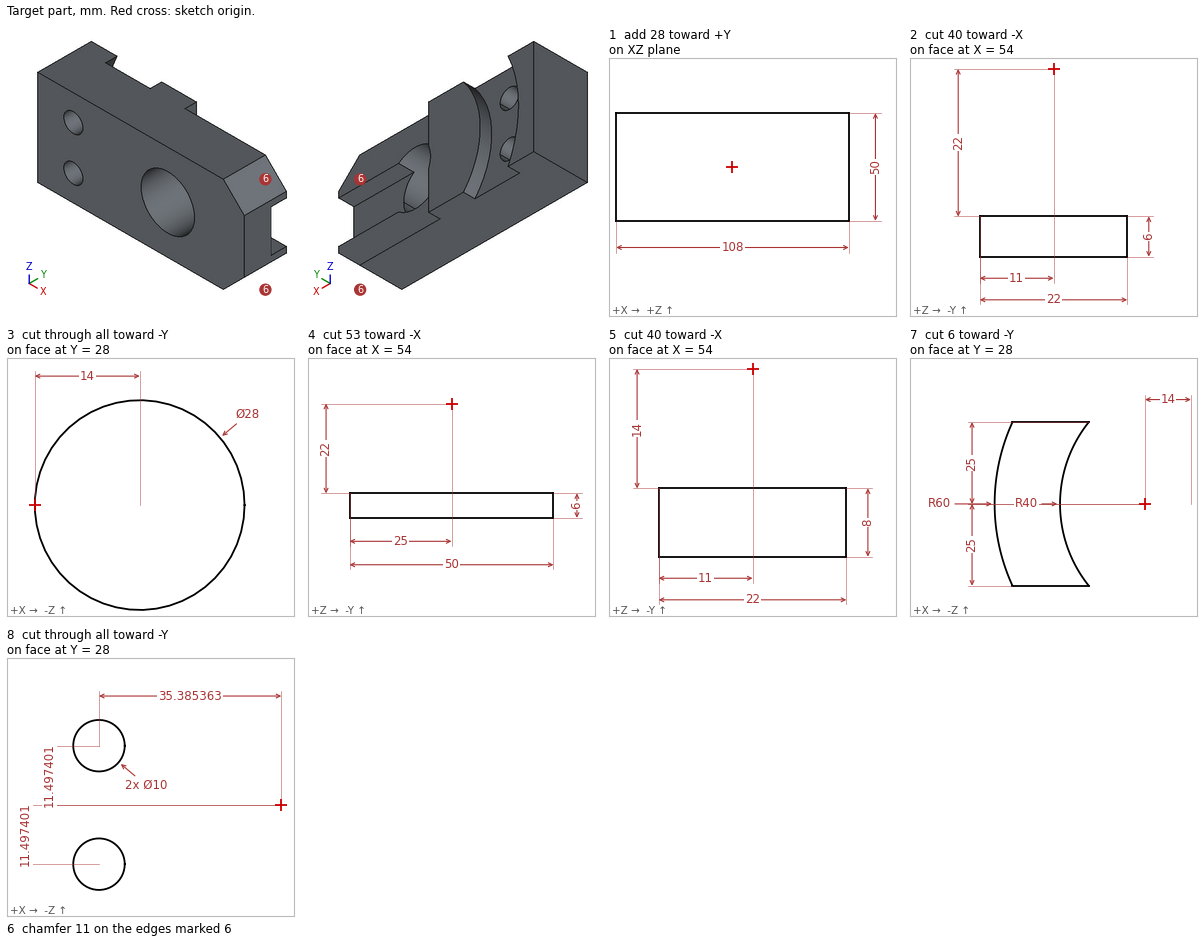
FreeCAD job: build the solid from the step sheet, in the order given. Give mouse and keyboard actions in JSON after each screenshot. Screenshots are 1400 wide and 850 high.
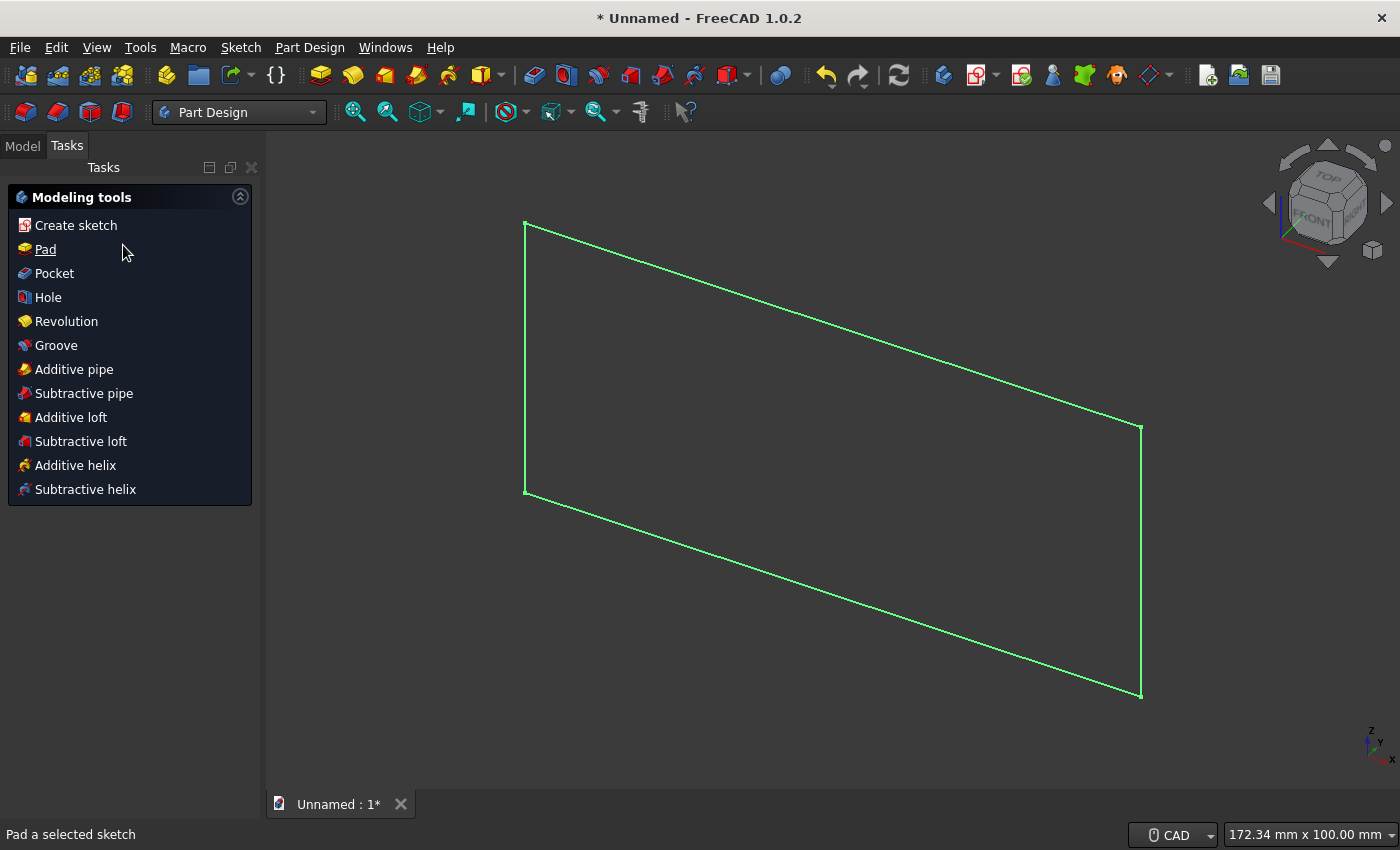
{"action": "left_click", "coordinate": [322, 76]}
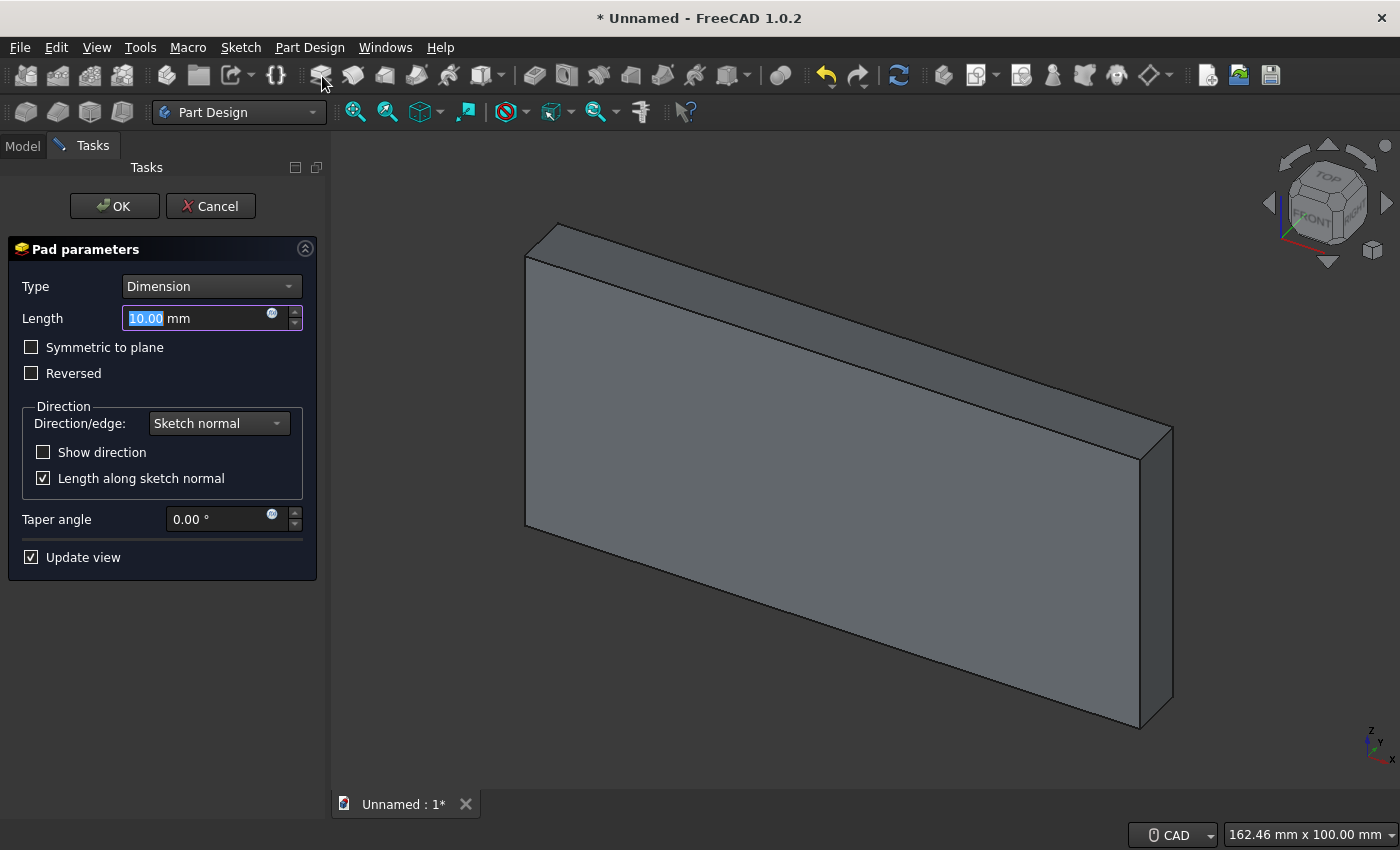
{"action": "type", "text": "28"}
{"action": "key", "text": "Tab"}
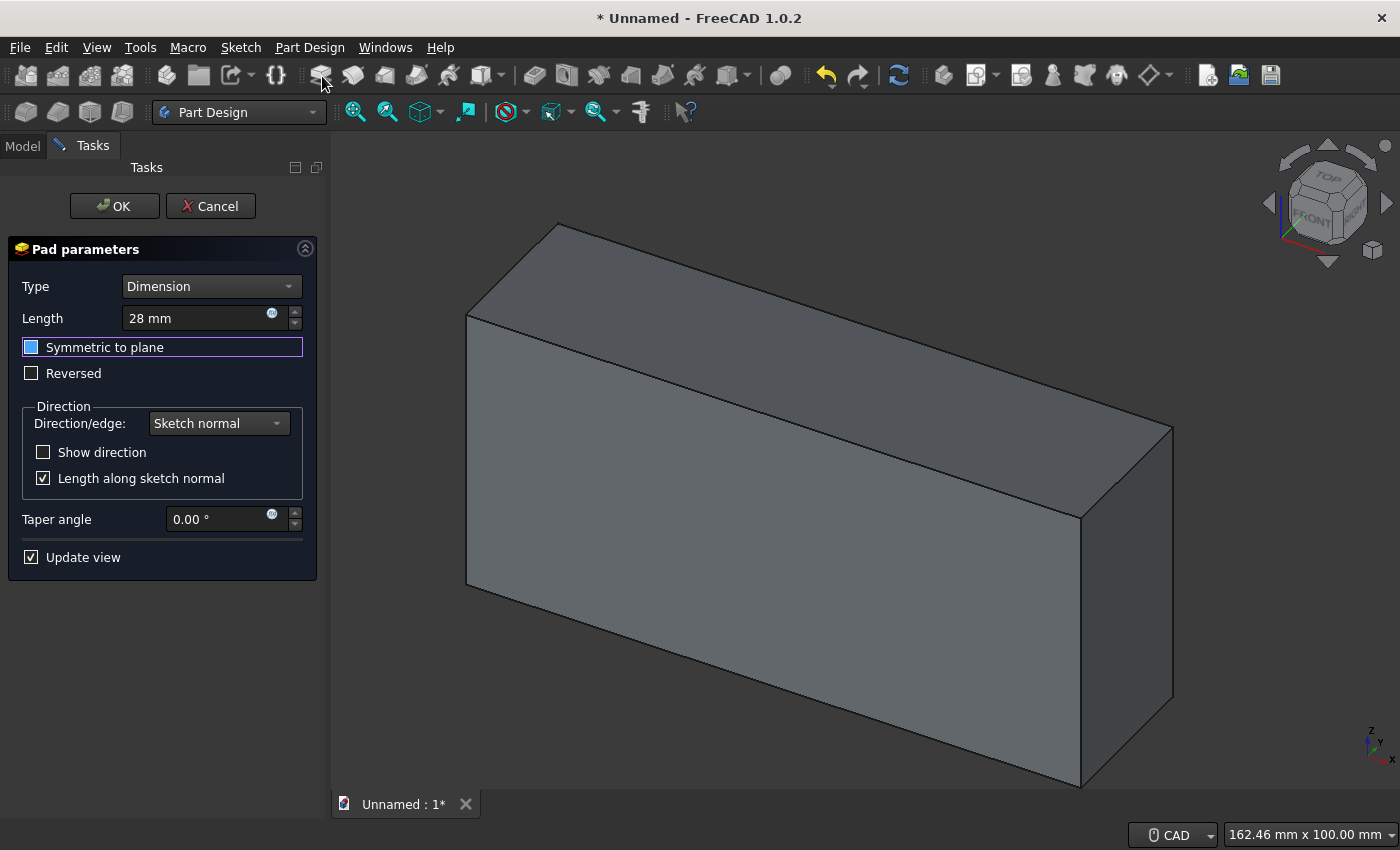
{"action": "left_click", "coordinate": [30, 373]}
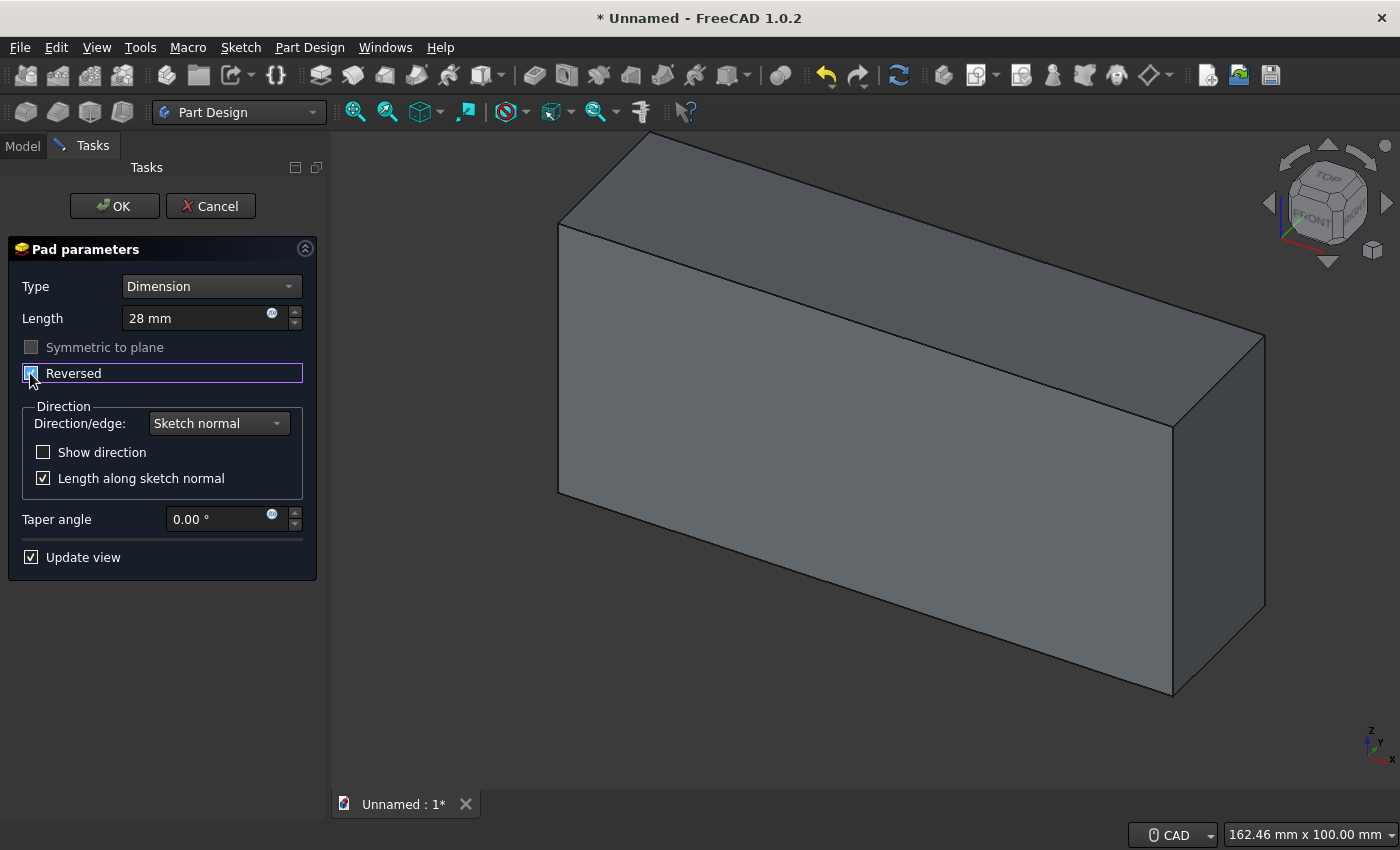
{"action": "left_click", "coordinate": [115, 206]}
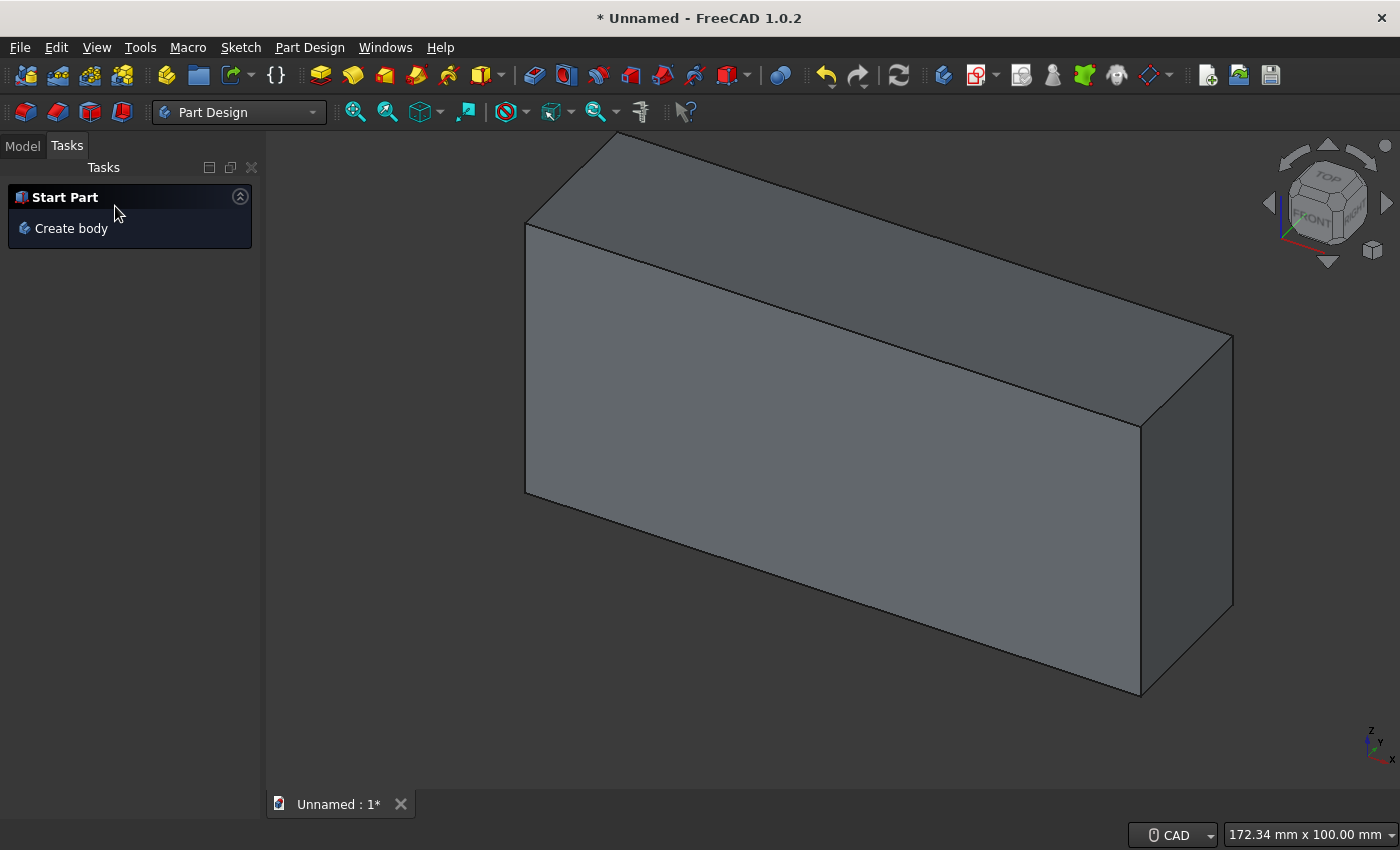
{"action": "left_click", "coordinate": [1187, 515]}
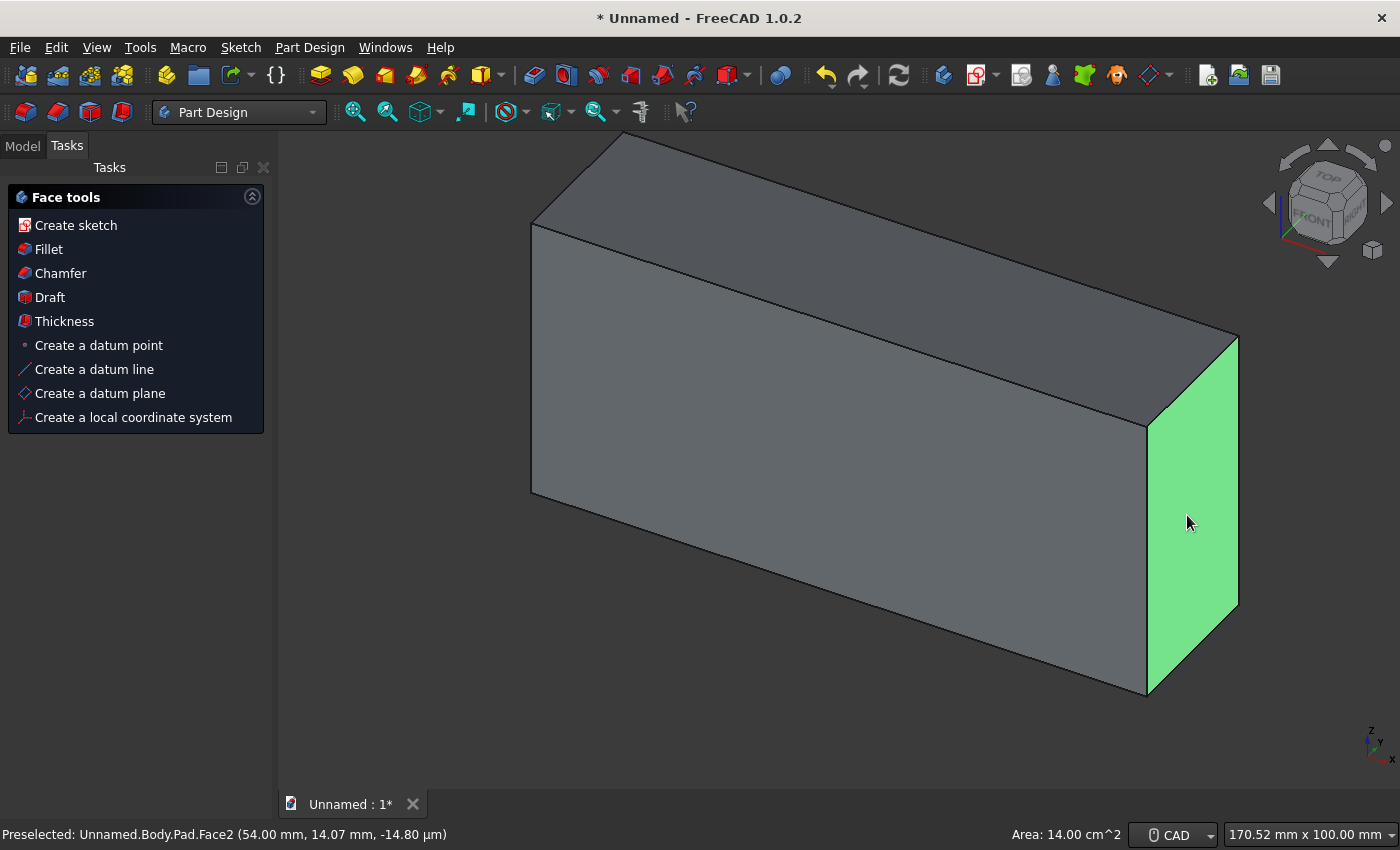
{"action": "left_click", "coordinate": [976, 76]}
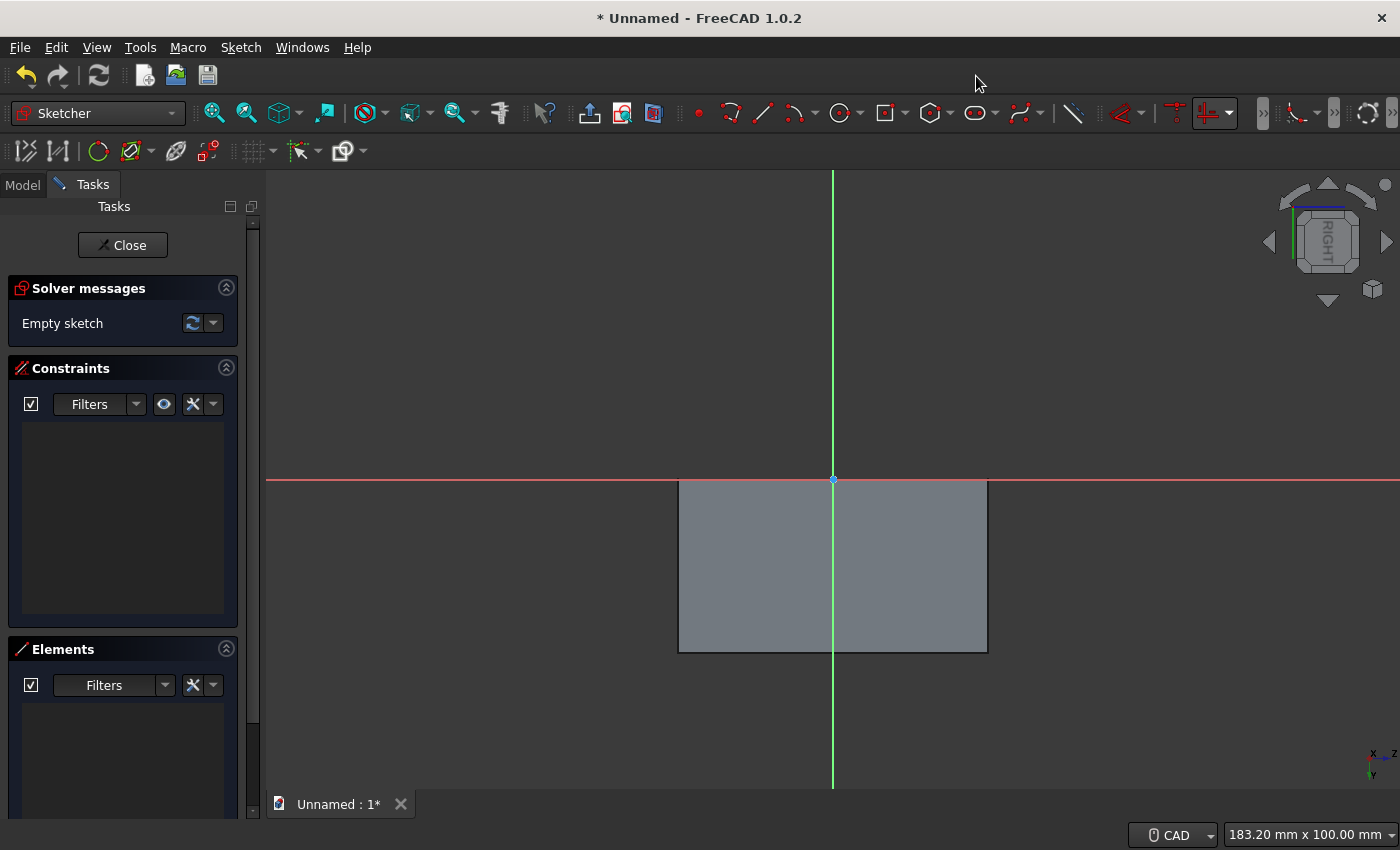
{"action": "scroll", "coordinate": [889, 637], "scroll_direction": "up", "scroll_amount": 4}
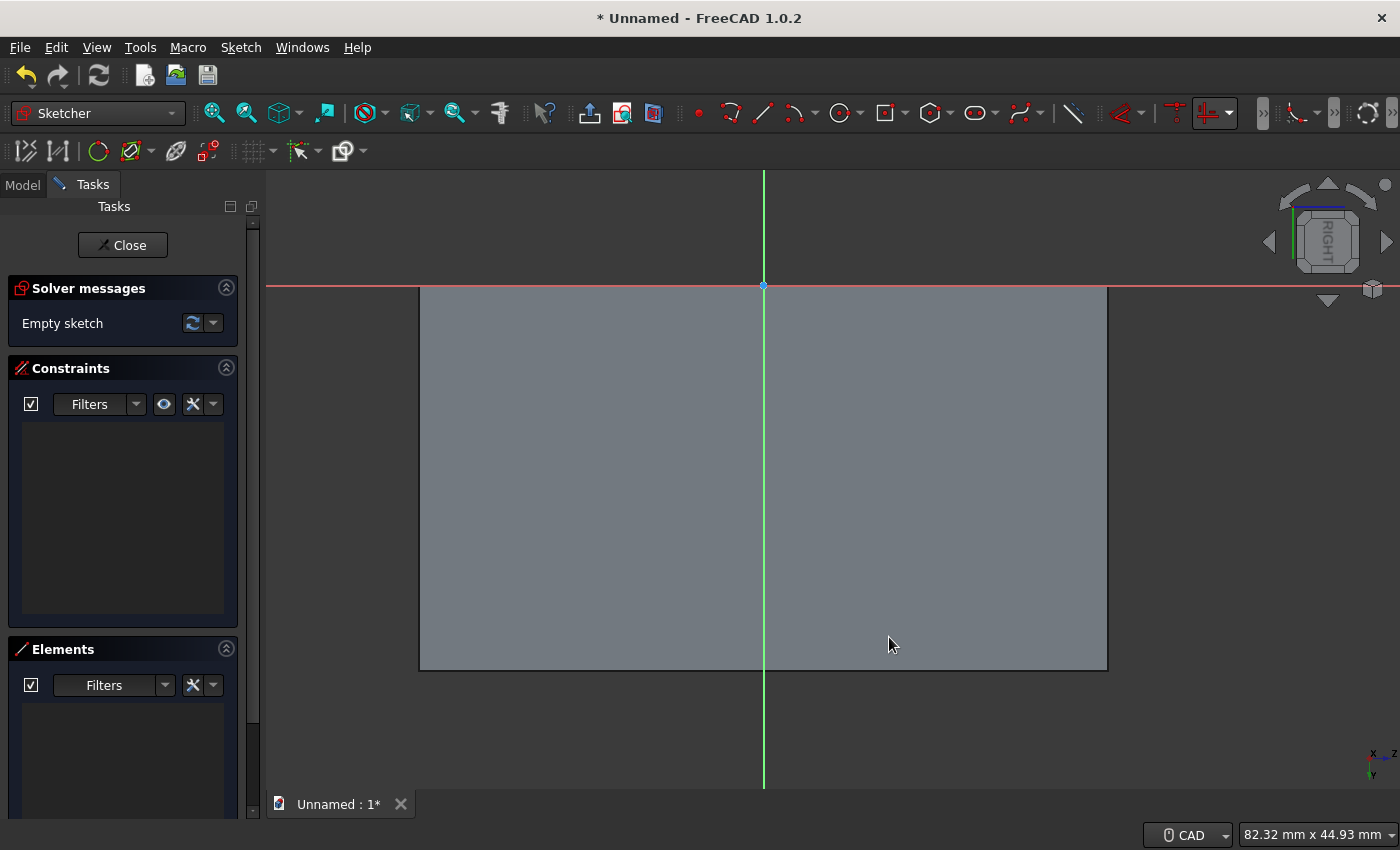
{"action": "left_click", "coordinate": [908, 114]}